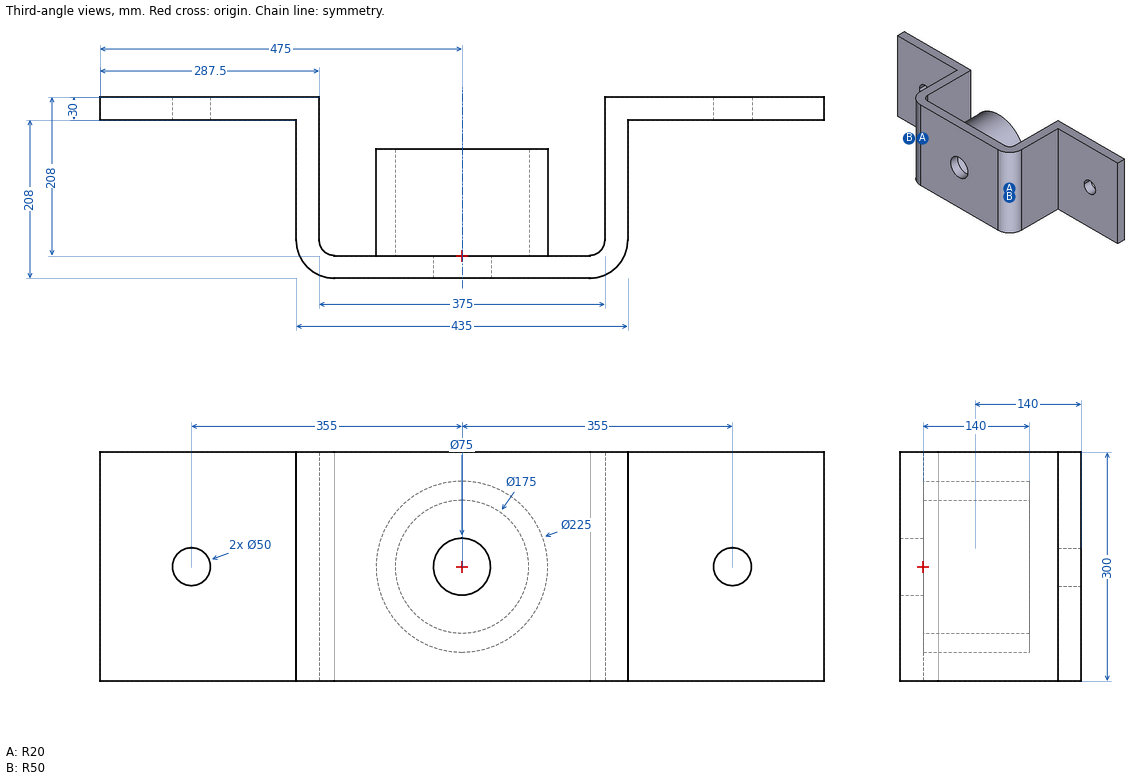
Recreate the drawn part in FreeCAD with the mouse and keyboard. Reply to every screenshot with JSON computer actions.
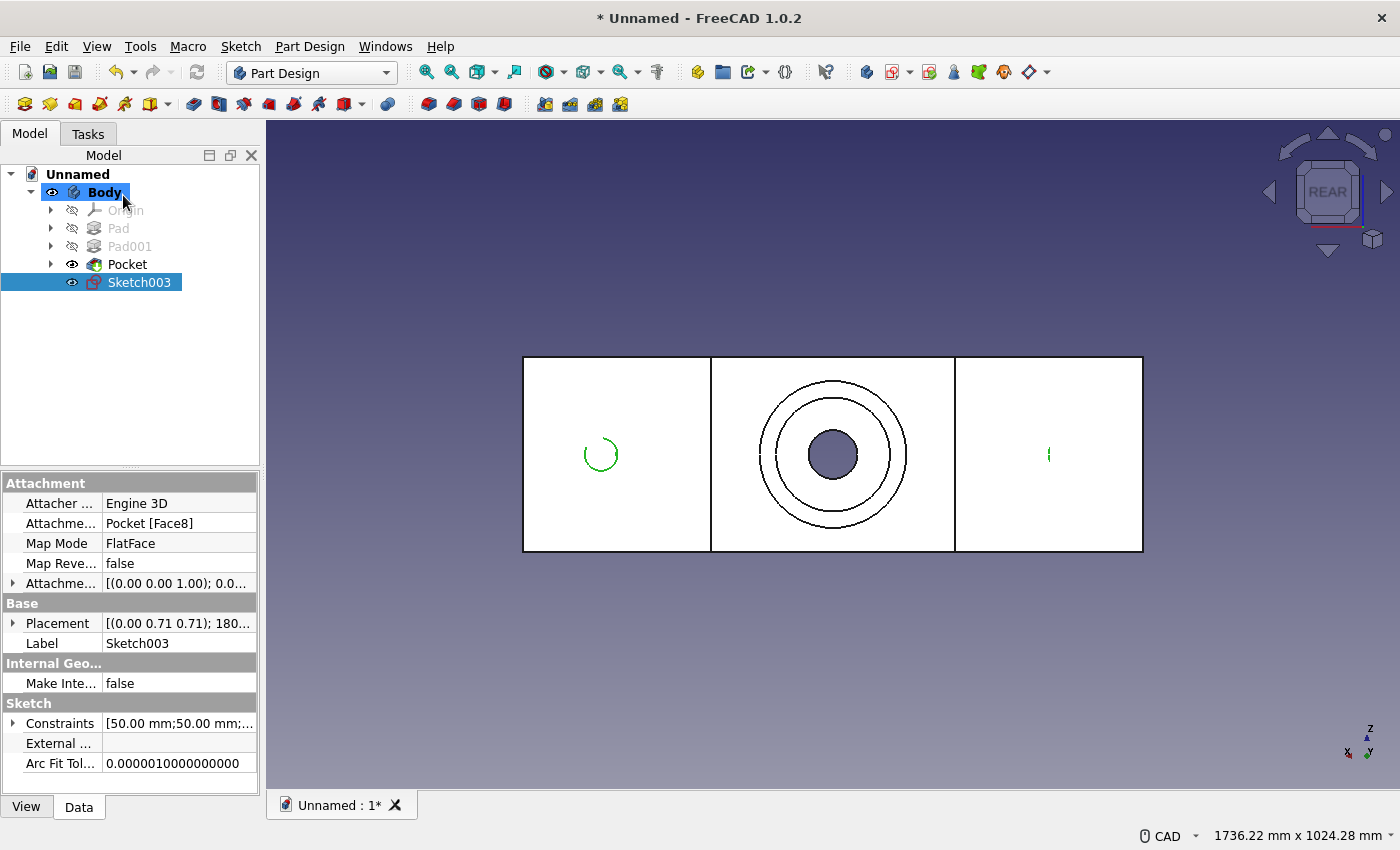
{"action": "left_click", "coordinate": [194, 104]}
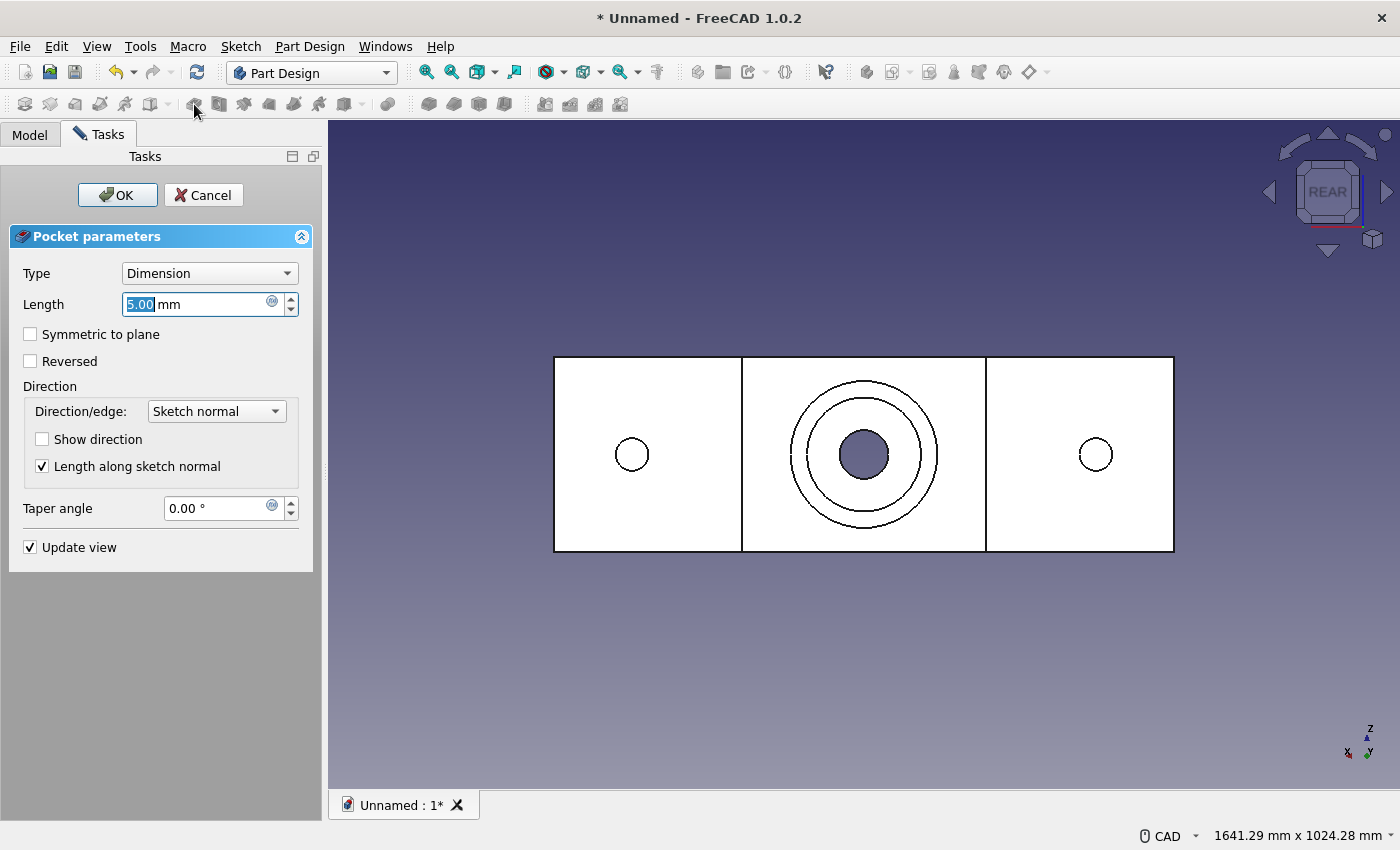
{"action": "type", "text": "140"}
{"action": "key", "text": "Tab"}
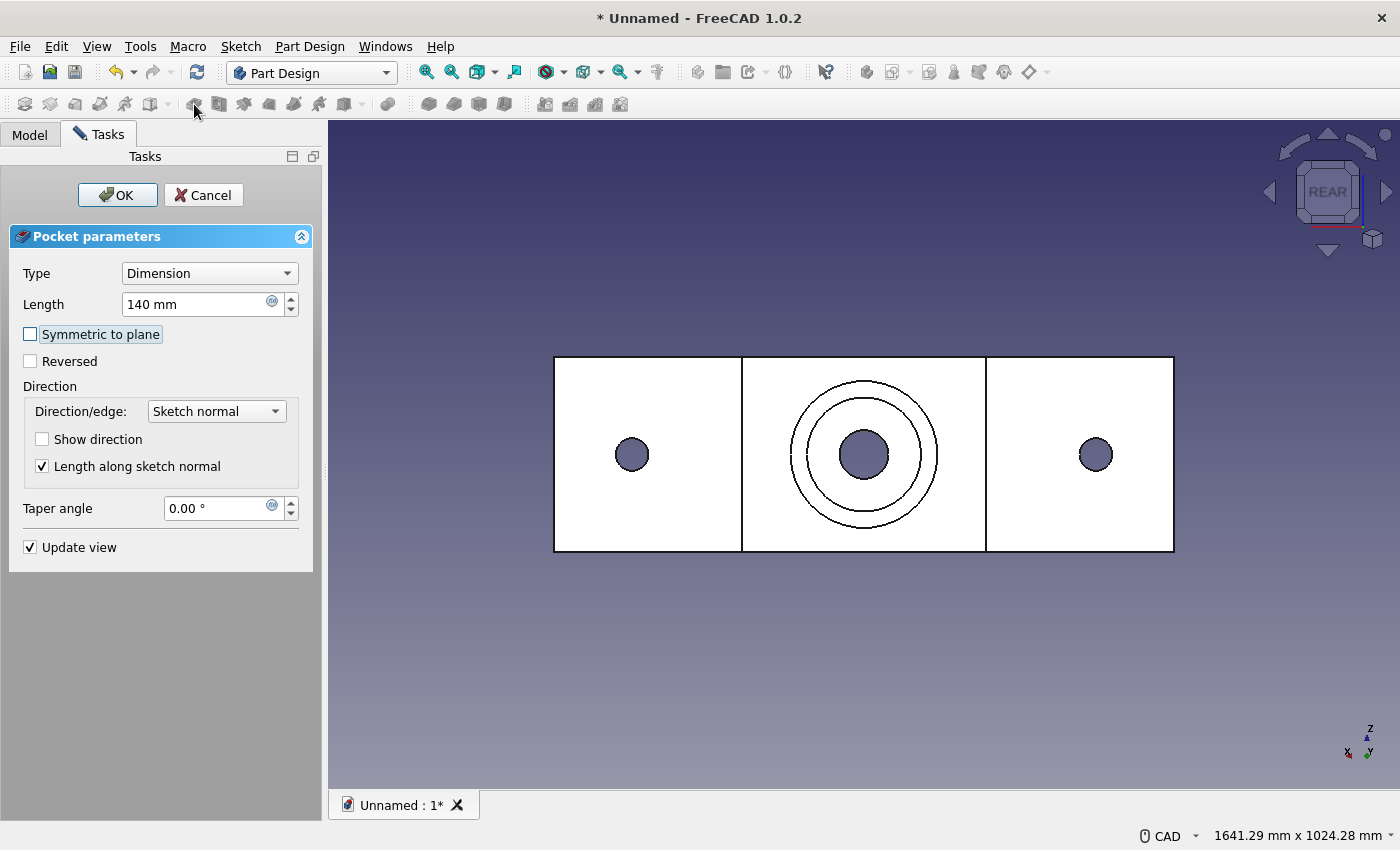
{"action": "left_click", "coordinate": [118, 195]}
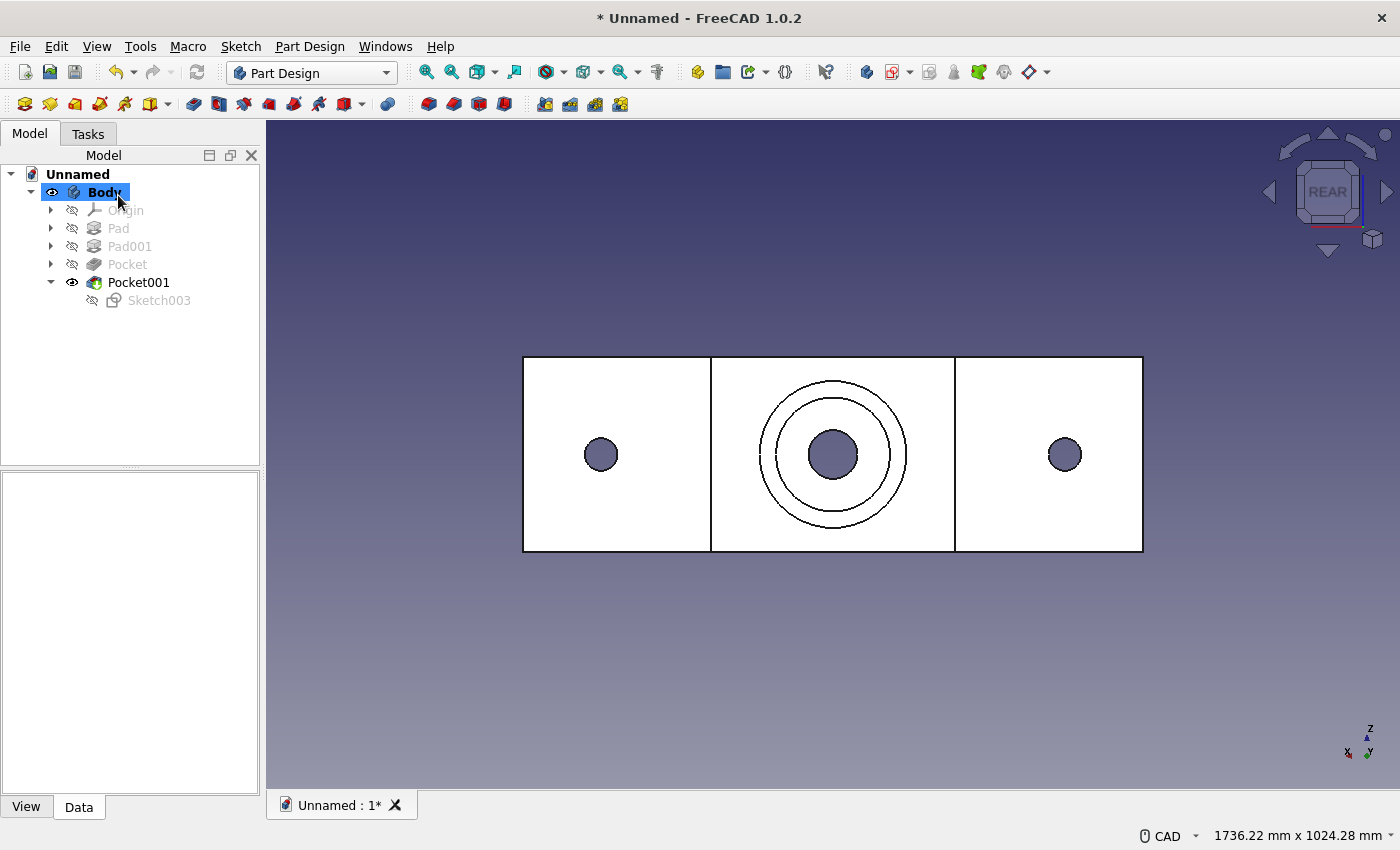
{"action": "key", "text": "0"}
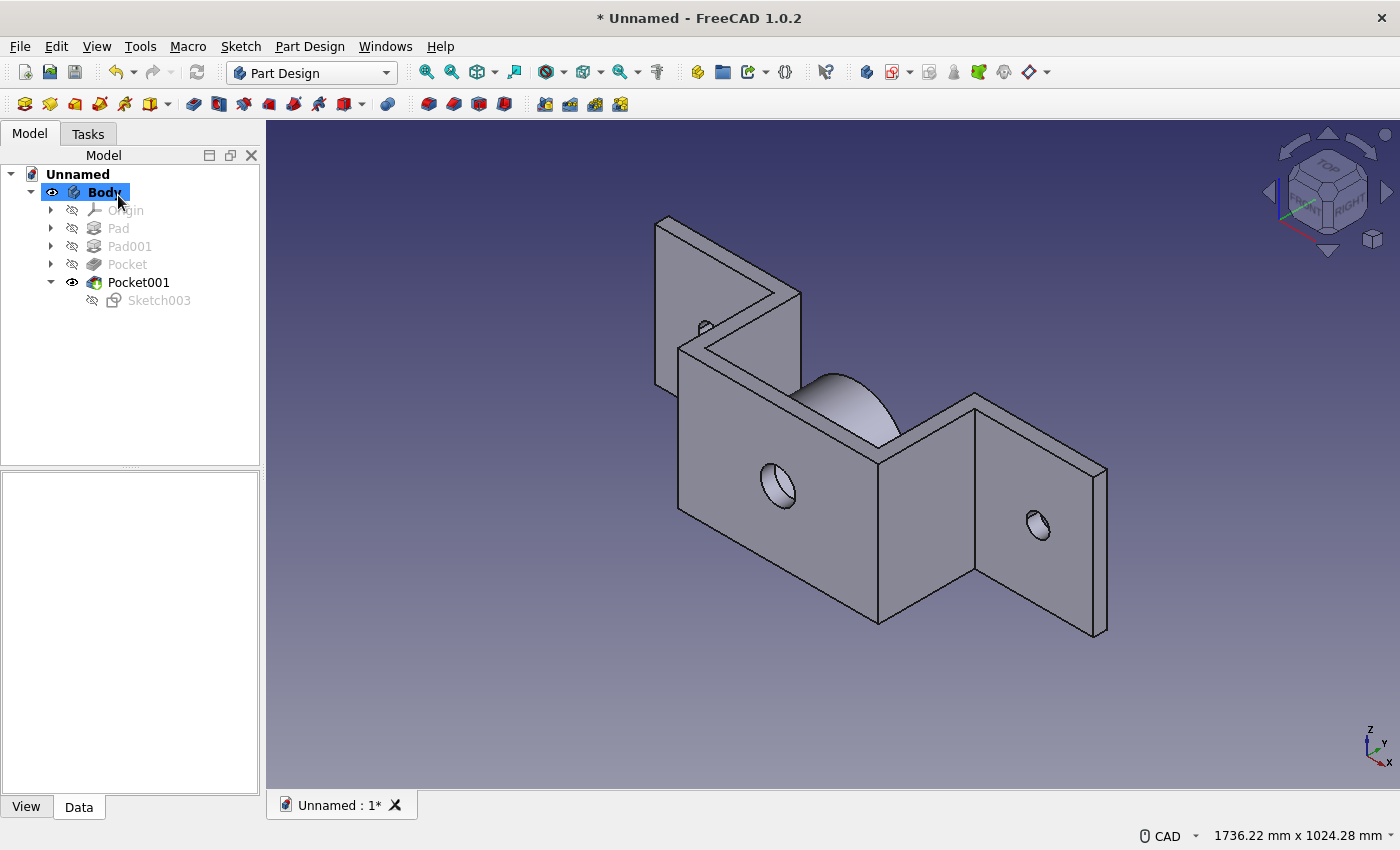
{"action": "key", "text": "2"}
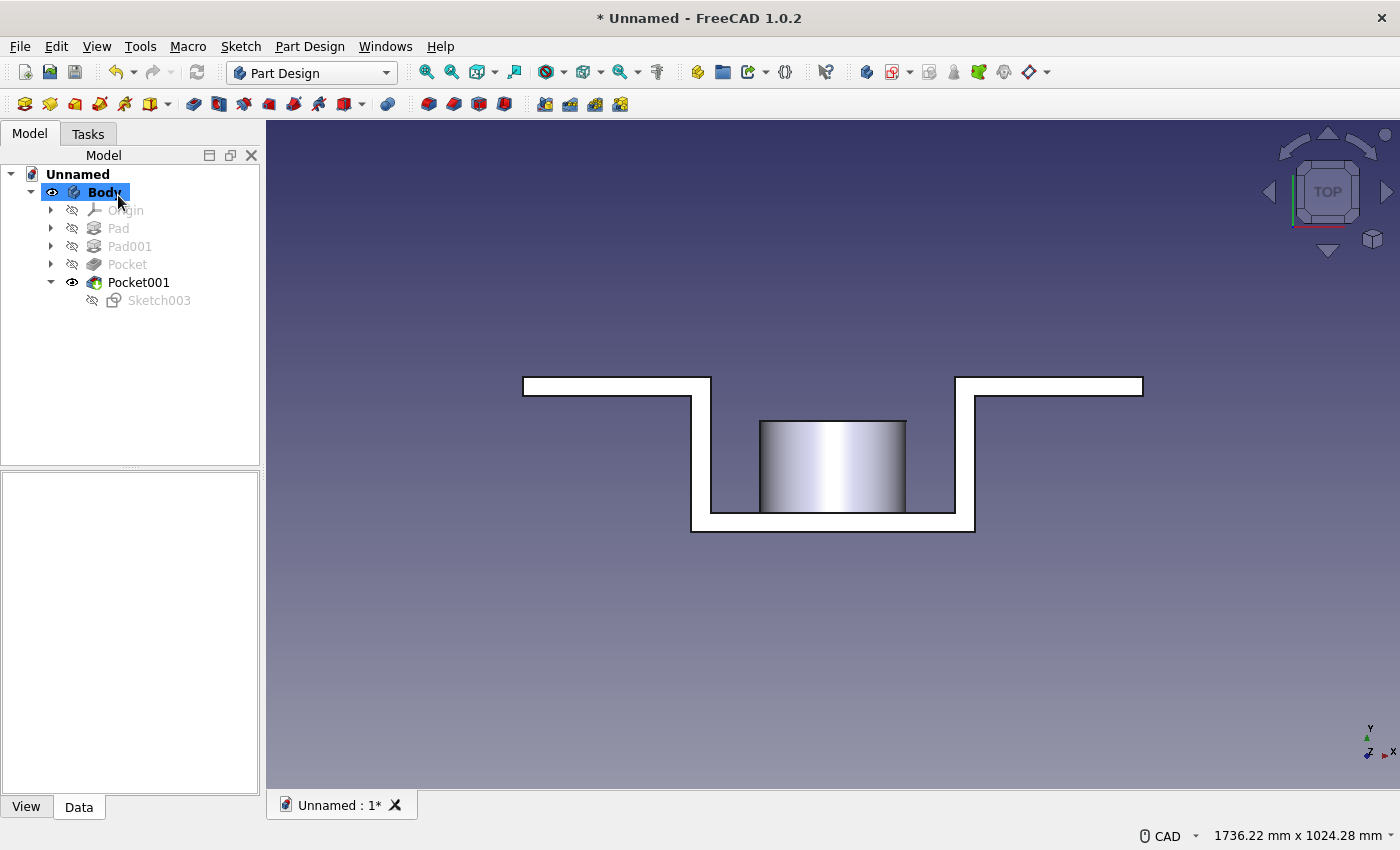
{"action": "key", "text": "1"}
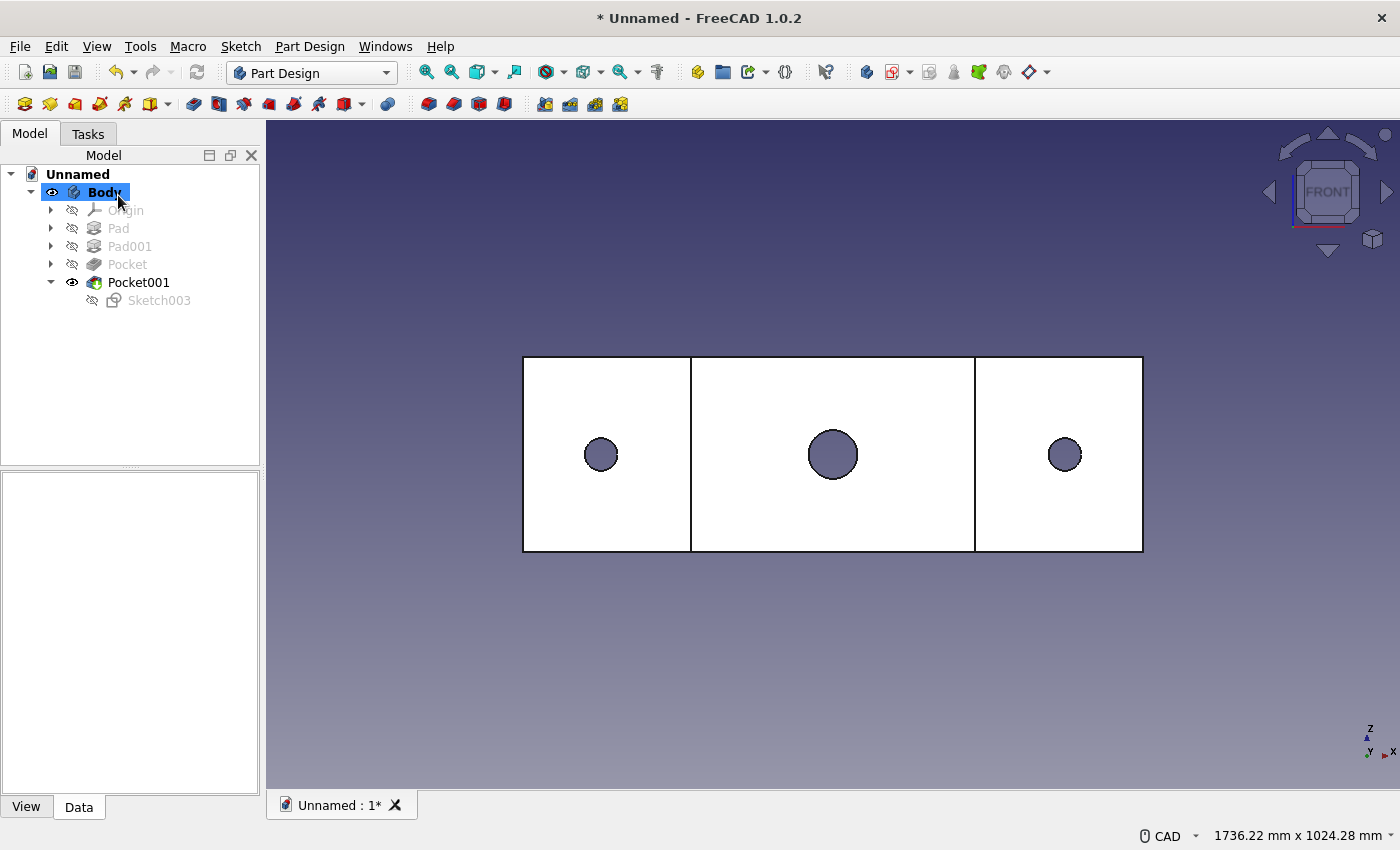
{"action": "key", "text": "3"}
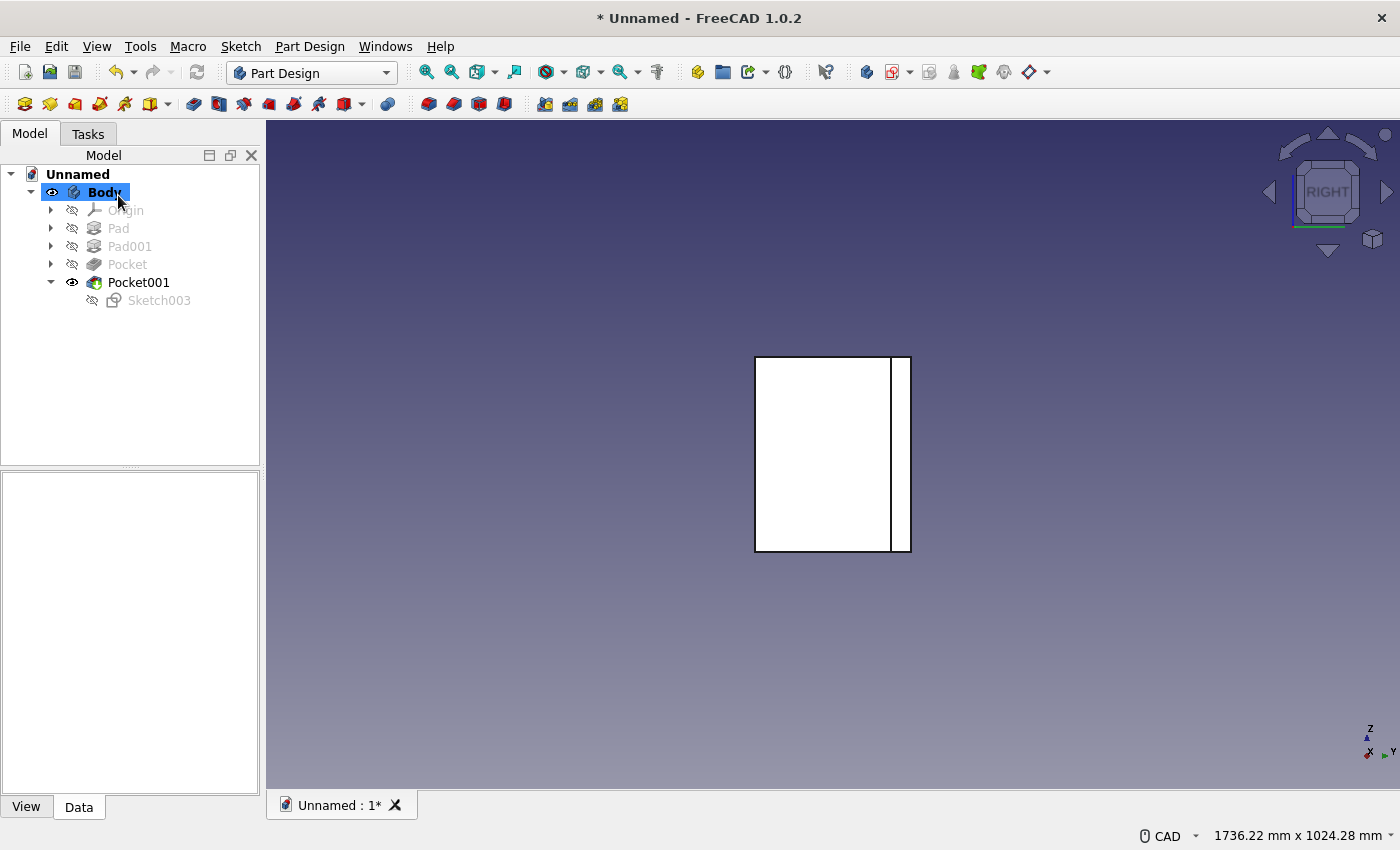
{"action": "left_click", "coordinate": [427, 72]}